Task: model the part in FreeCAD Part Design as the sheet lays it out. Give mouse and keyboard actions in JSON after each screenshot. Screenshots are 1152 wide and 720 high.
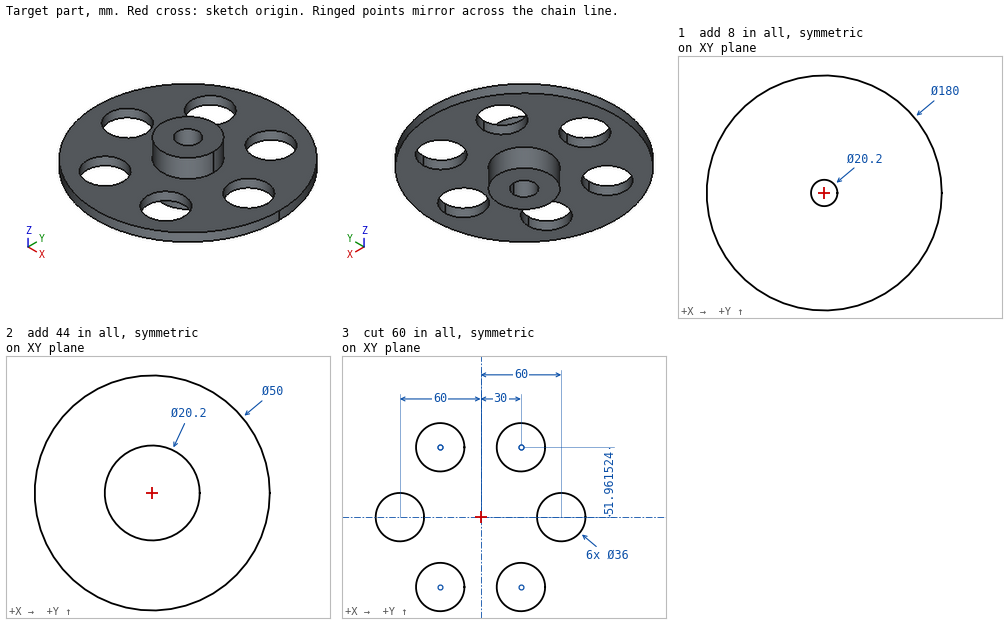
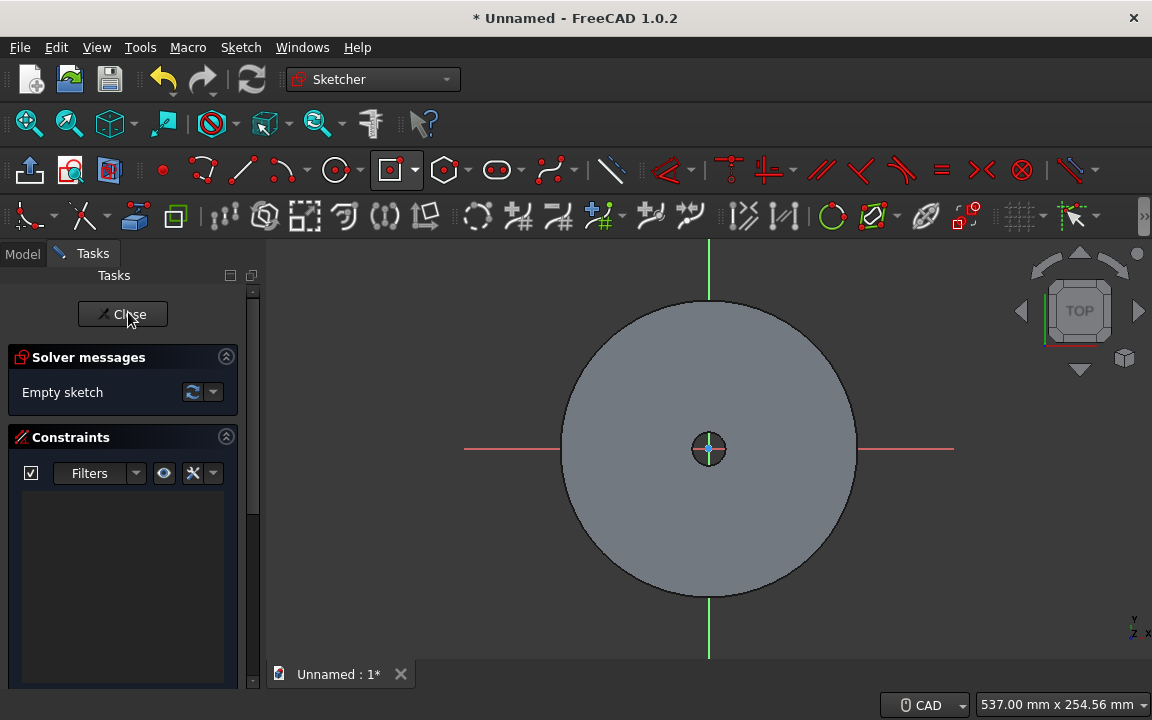
{"action": "left_click", "coordinate": [110, 170]}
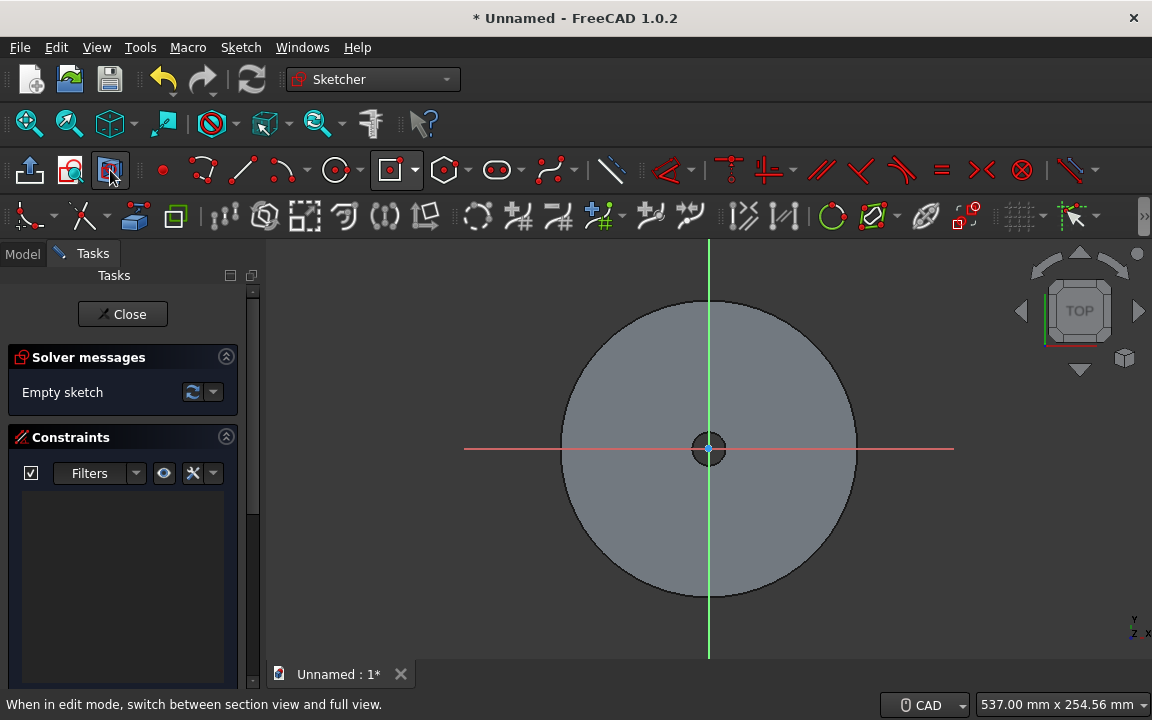
{"action": "scroll", "coordinate": [738, 449], "scroll_direction": "up", "scroll_amount": 6}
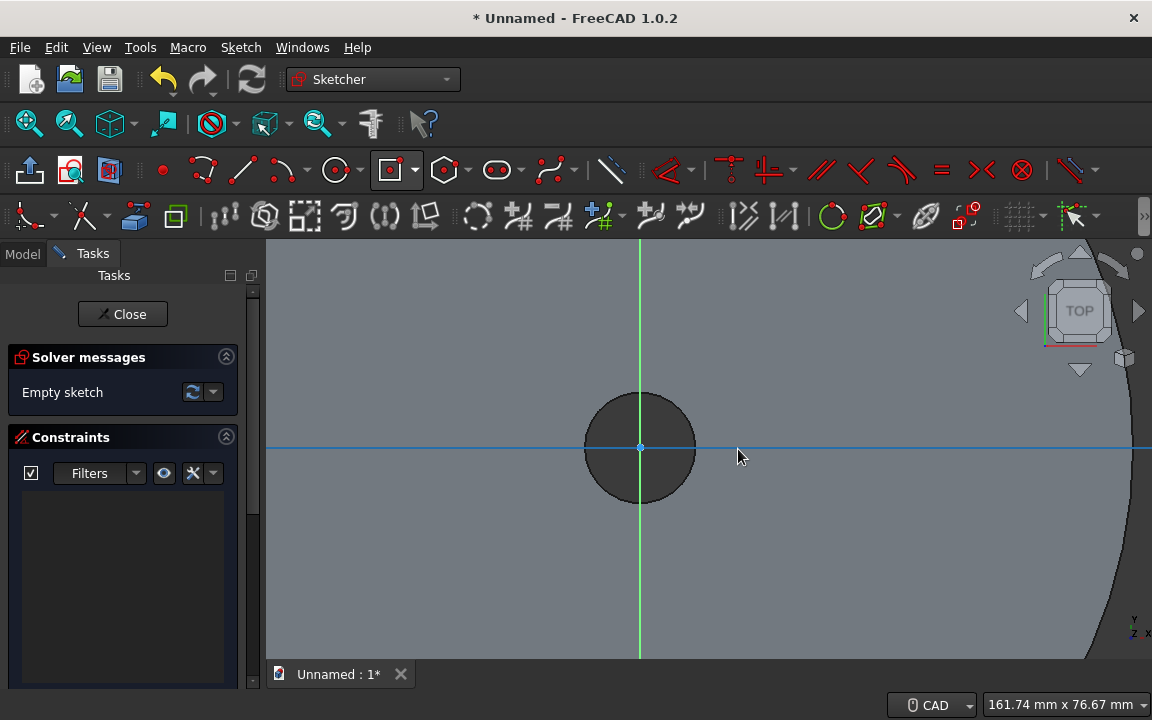
{"action": "left_click", "coordinate": [336, 170]}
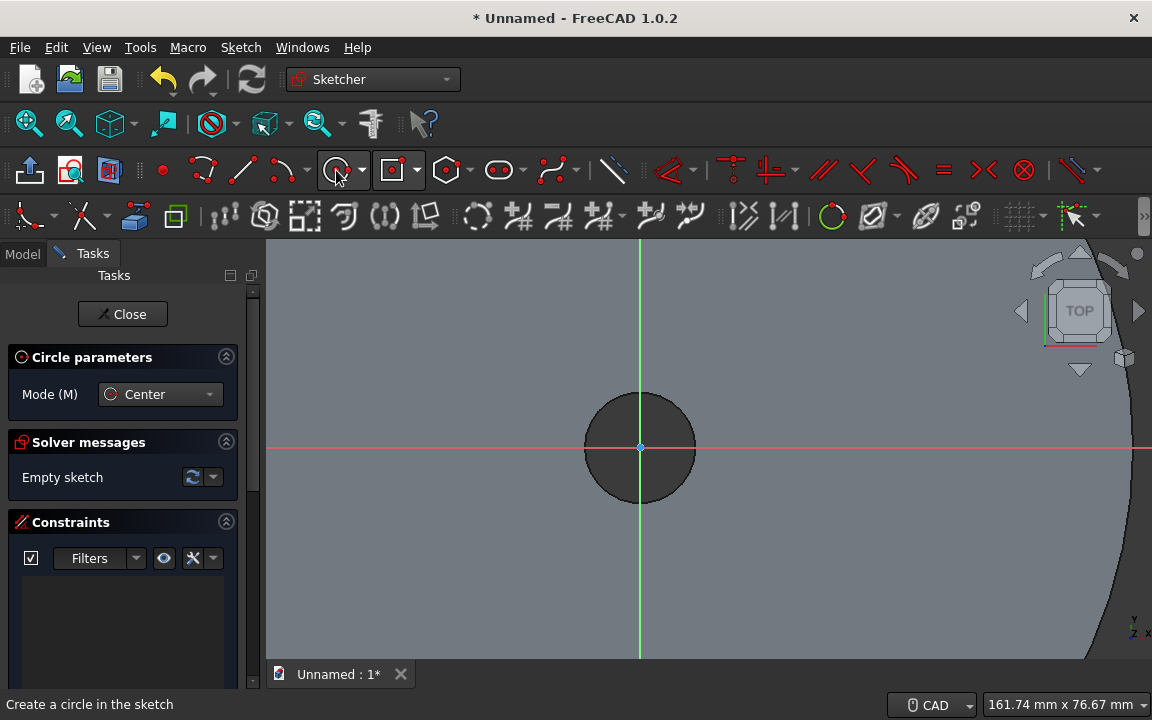
{"action": "left_click", "coordinate": [640, 448]}
{"action": "left_click", "coordinate": [737, 351]}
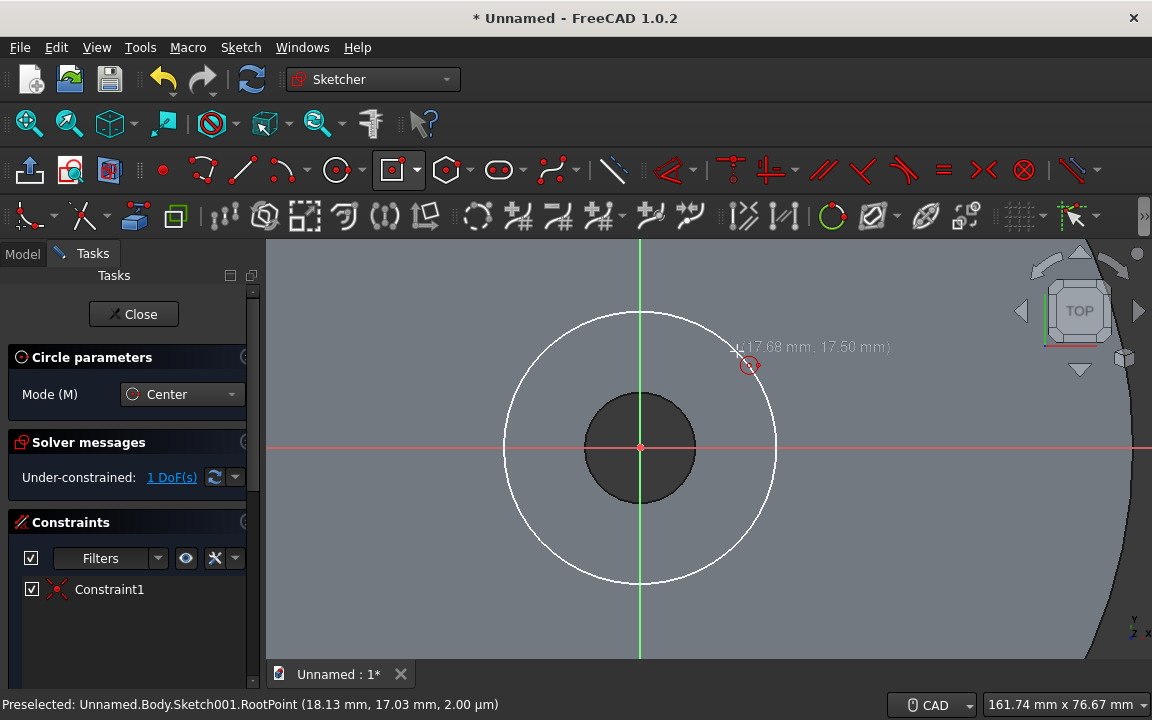
{"action": "left_click", "coordinate": [640, 448]}
{"action": "left_click", "coordinate": [679, 409]}
{"action": "key", "text": "Escape"}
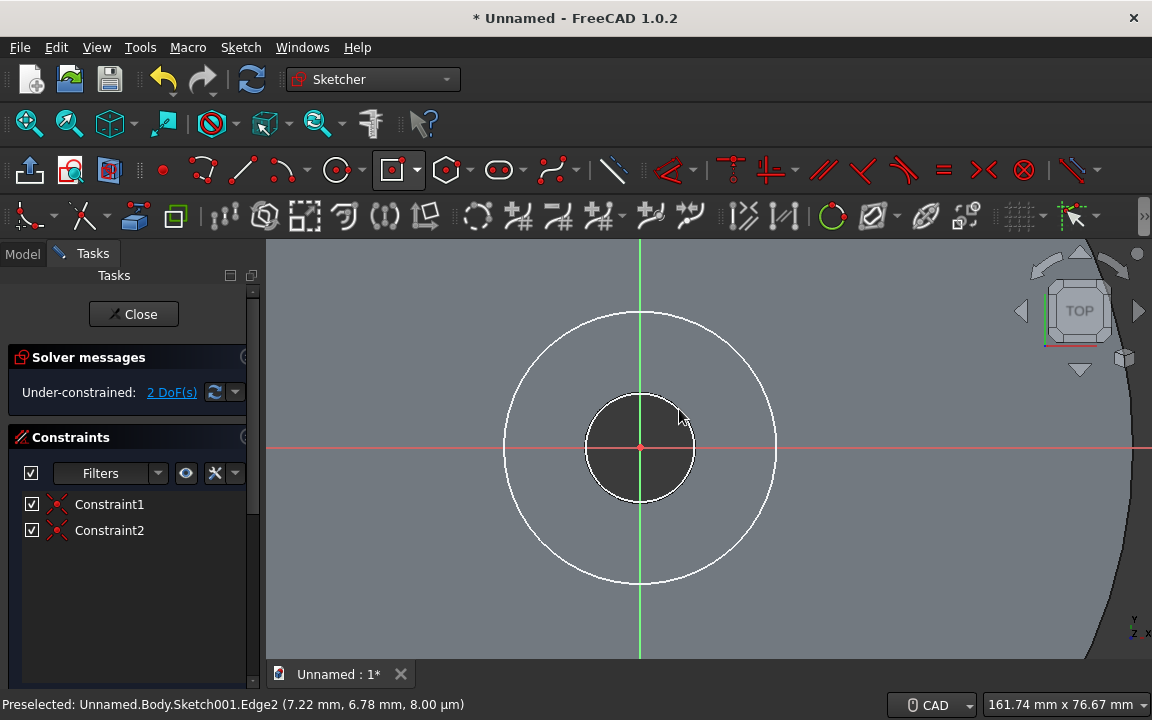
{"action": "left_click", "coordinate": [736, 351]}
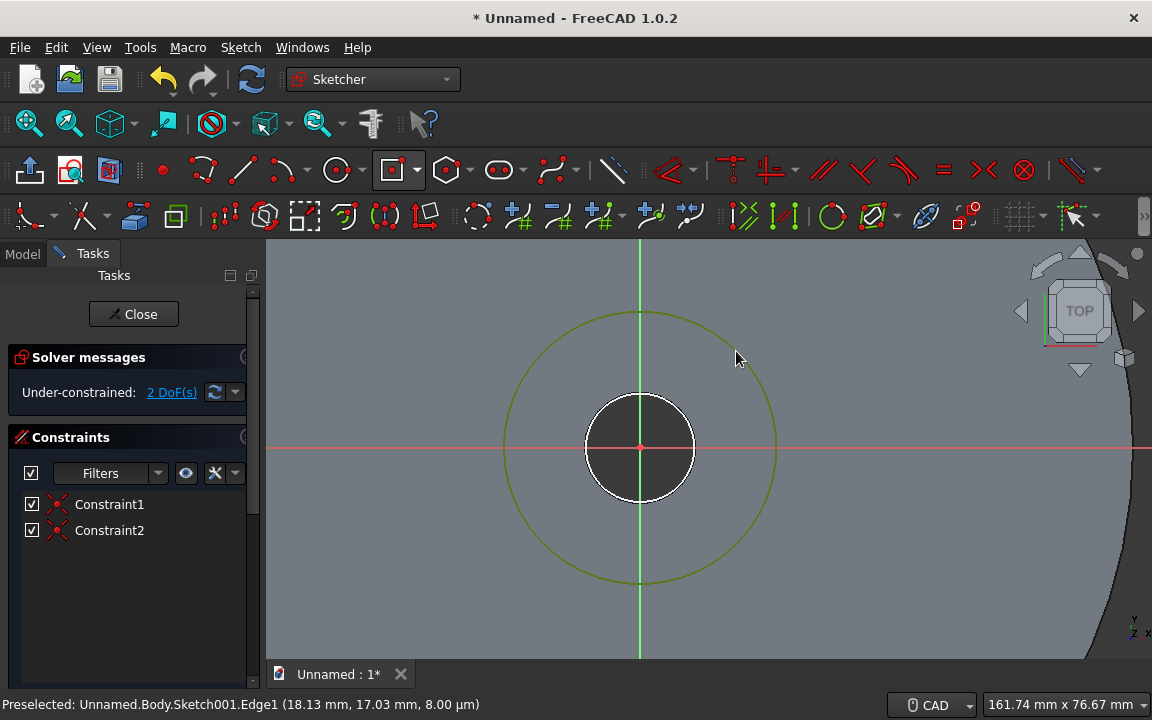
{"action": "left_click", "coordinate": [696, 170]}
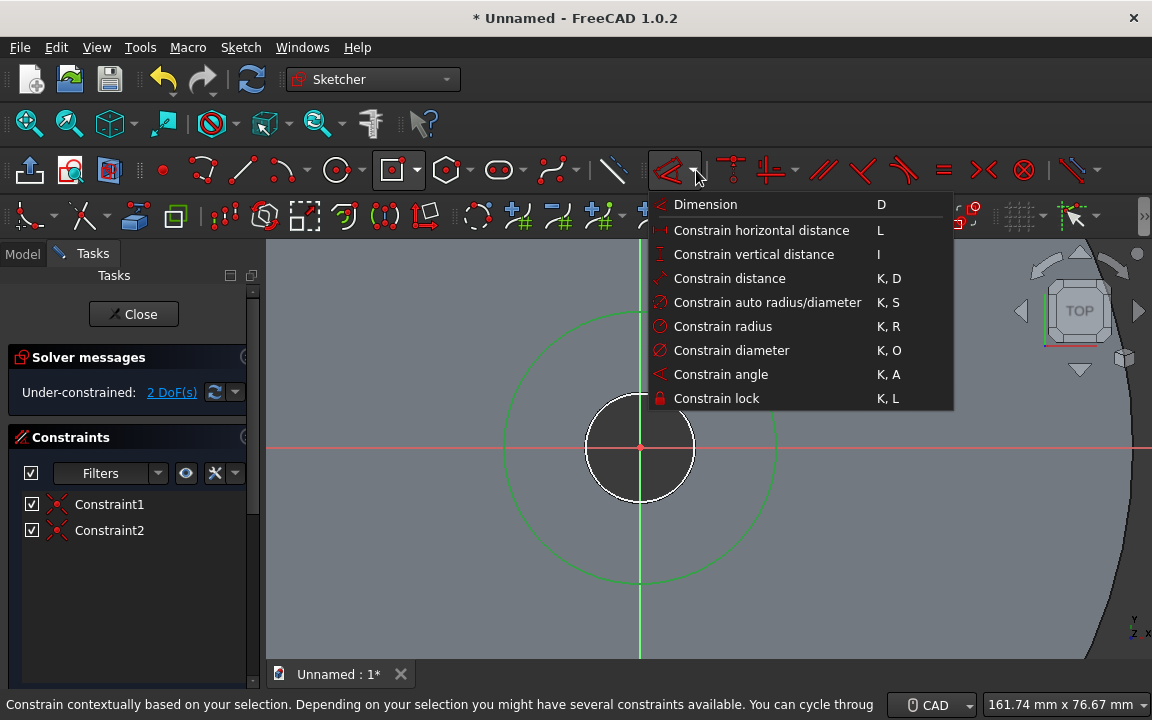
{"action": "left_click", "coordinate": [801, 350]}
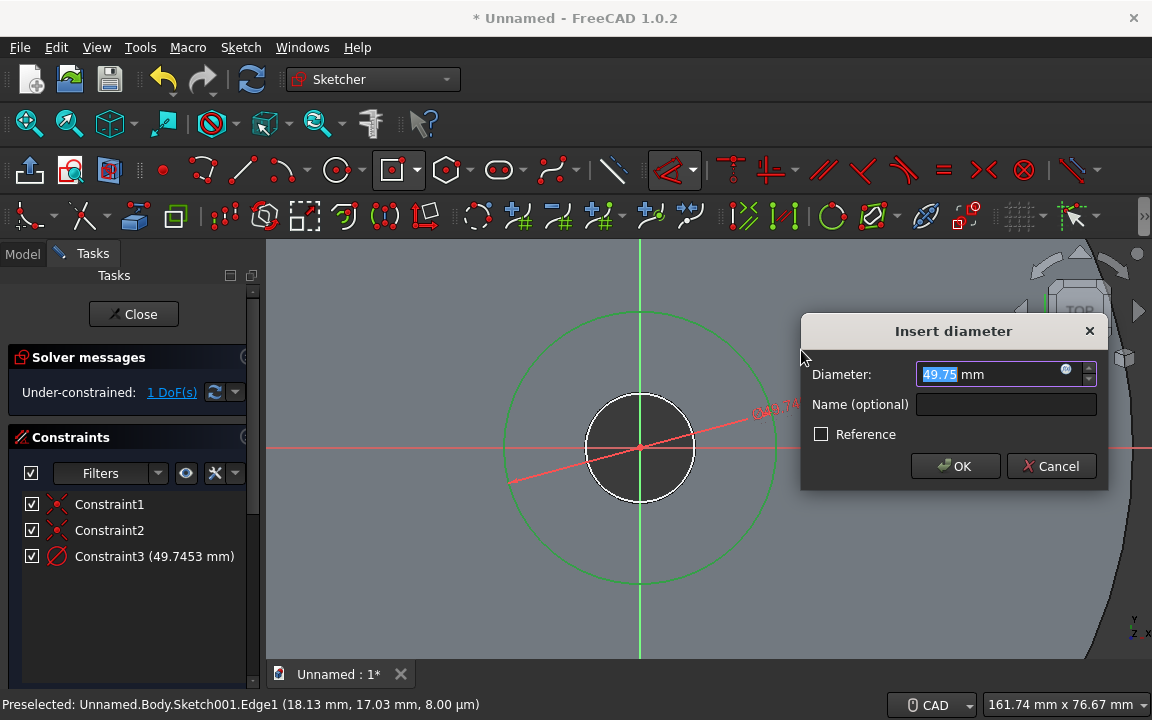
{"action": "type", "text": "50"}
{"action": "key", "text": "Return"}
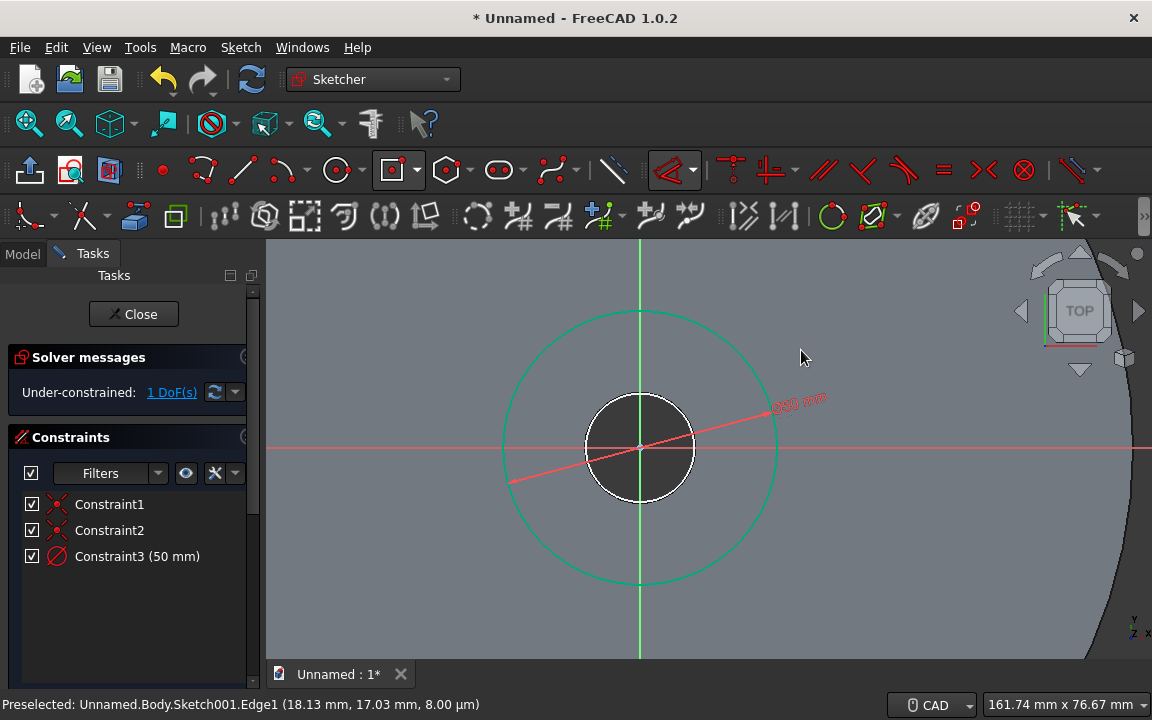
{"action": "left_click", "coordinate": [678, 409]}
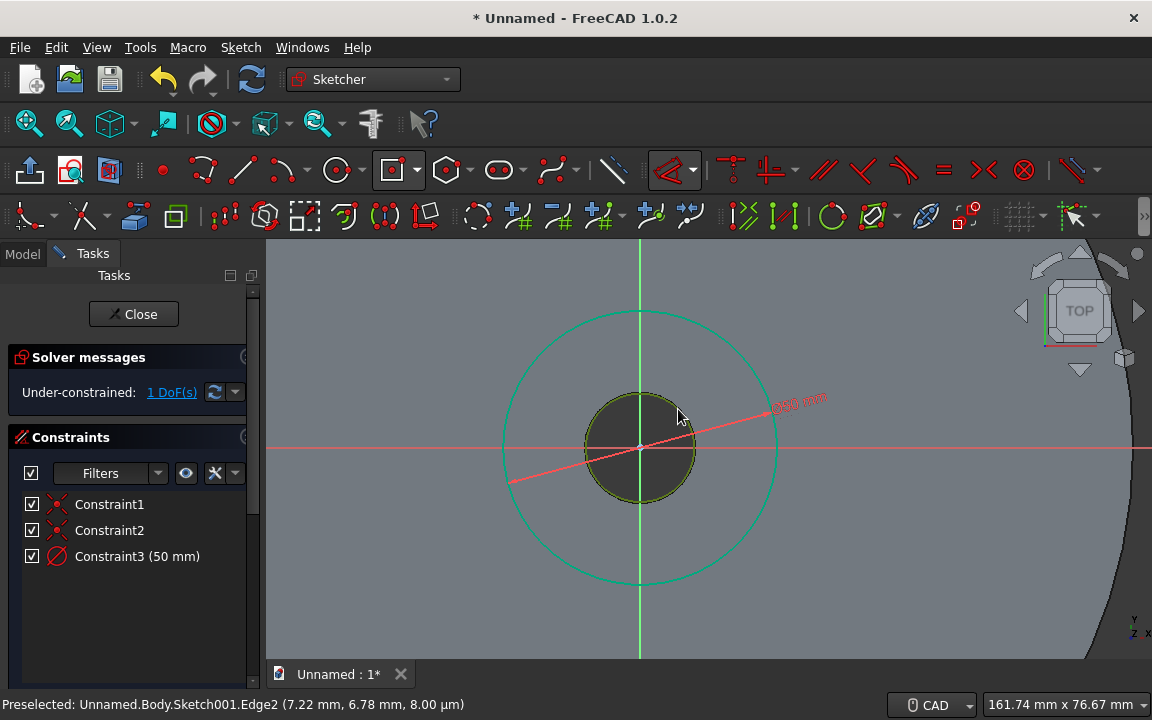
{"action": "key", "text": "k o"}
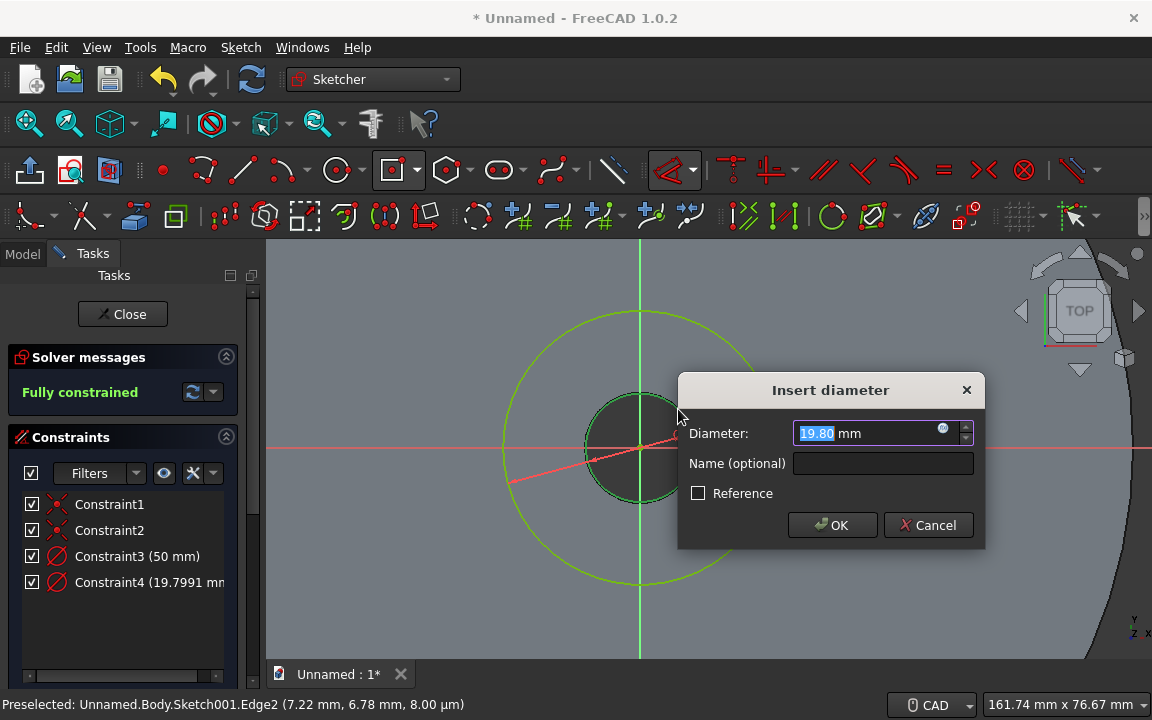
{"action": "type", "text": "20.2"}
{"action": "key", "text": "Return"}